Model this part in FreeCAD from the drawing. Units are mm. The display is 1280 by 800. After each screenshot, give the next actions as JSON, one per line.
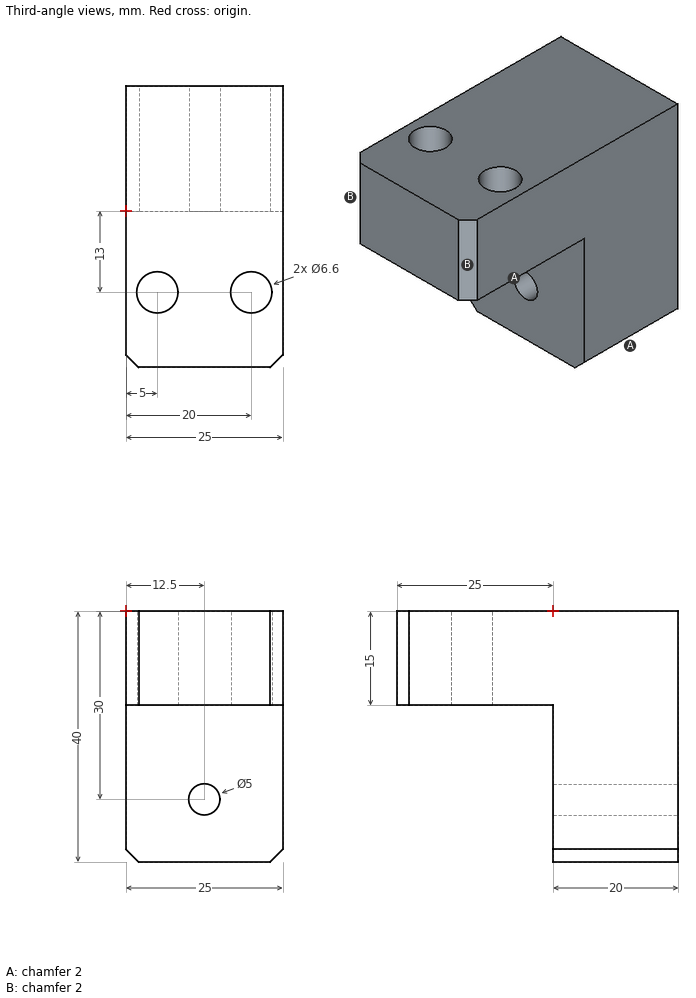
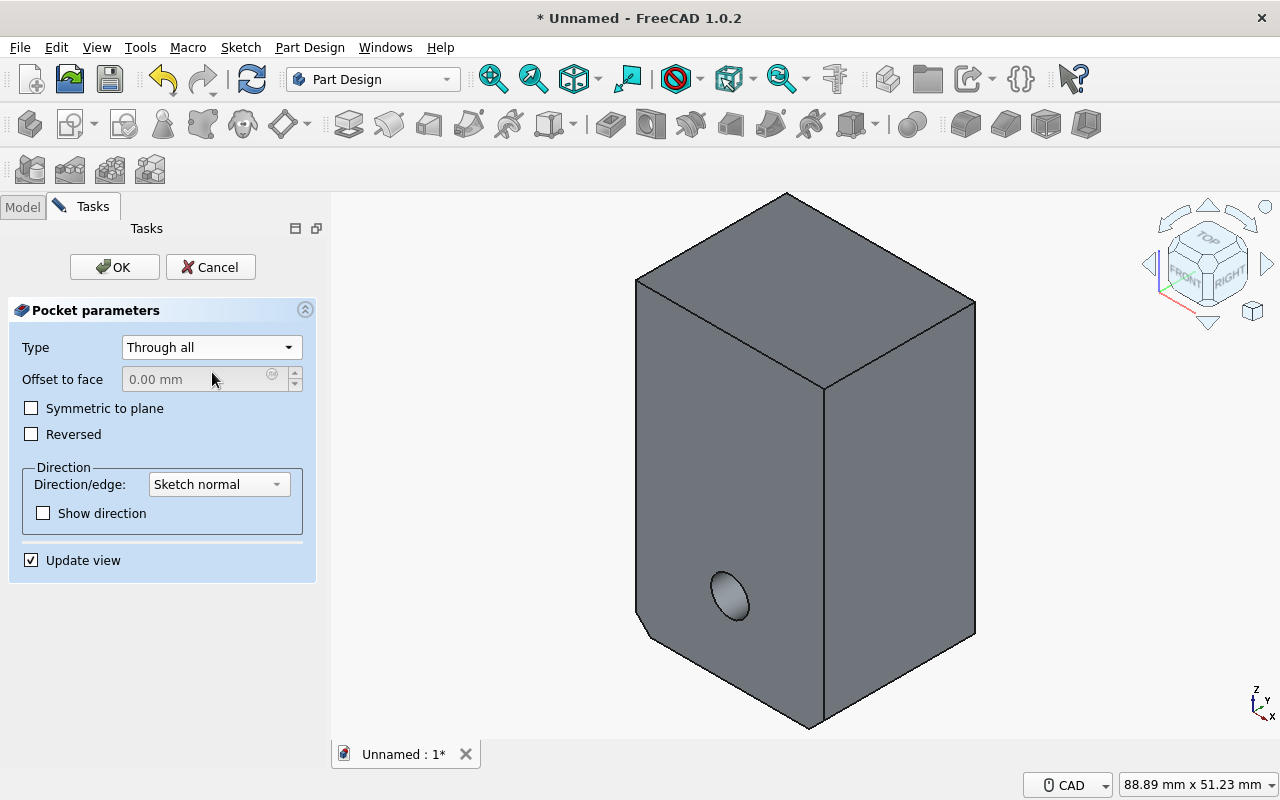
{"action": "left_click", "coordinate": [115, 267]}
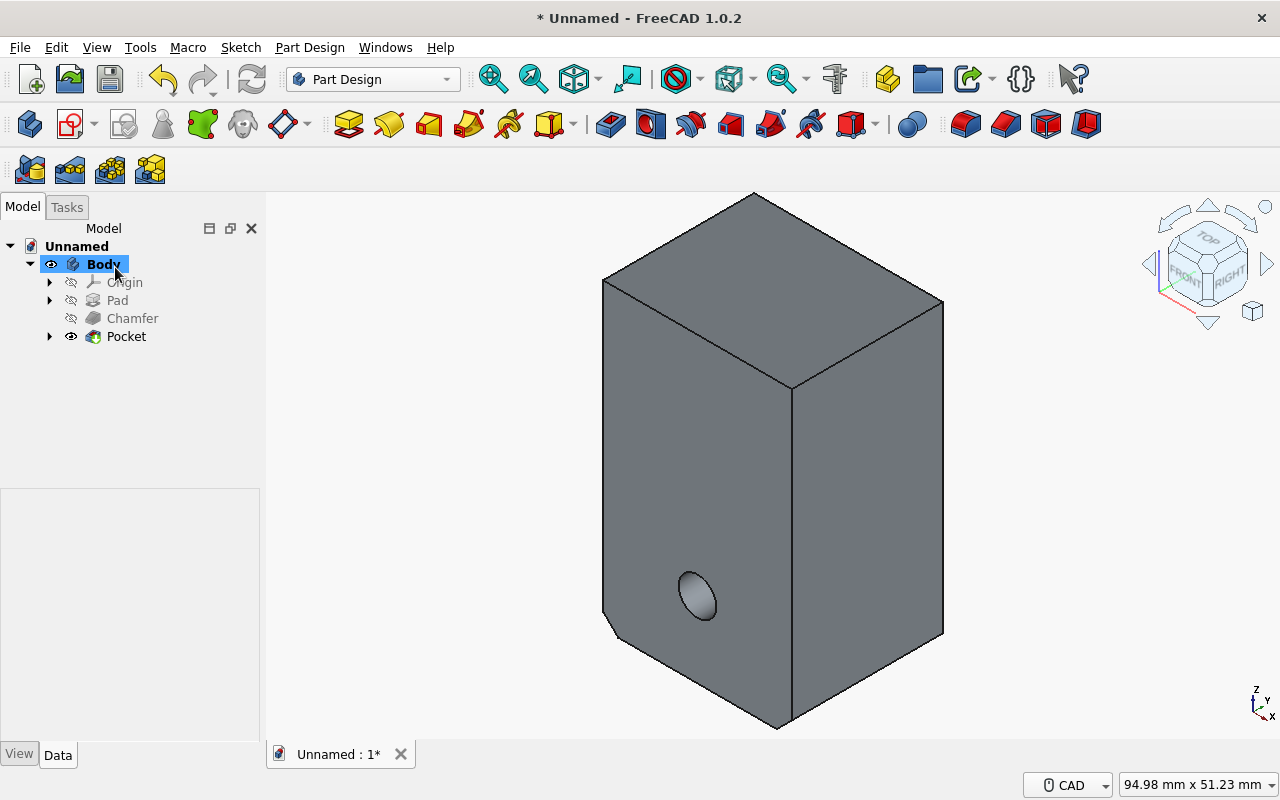
{"action": "left_click", "coordinate": [867, 463]}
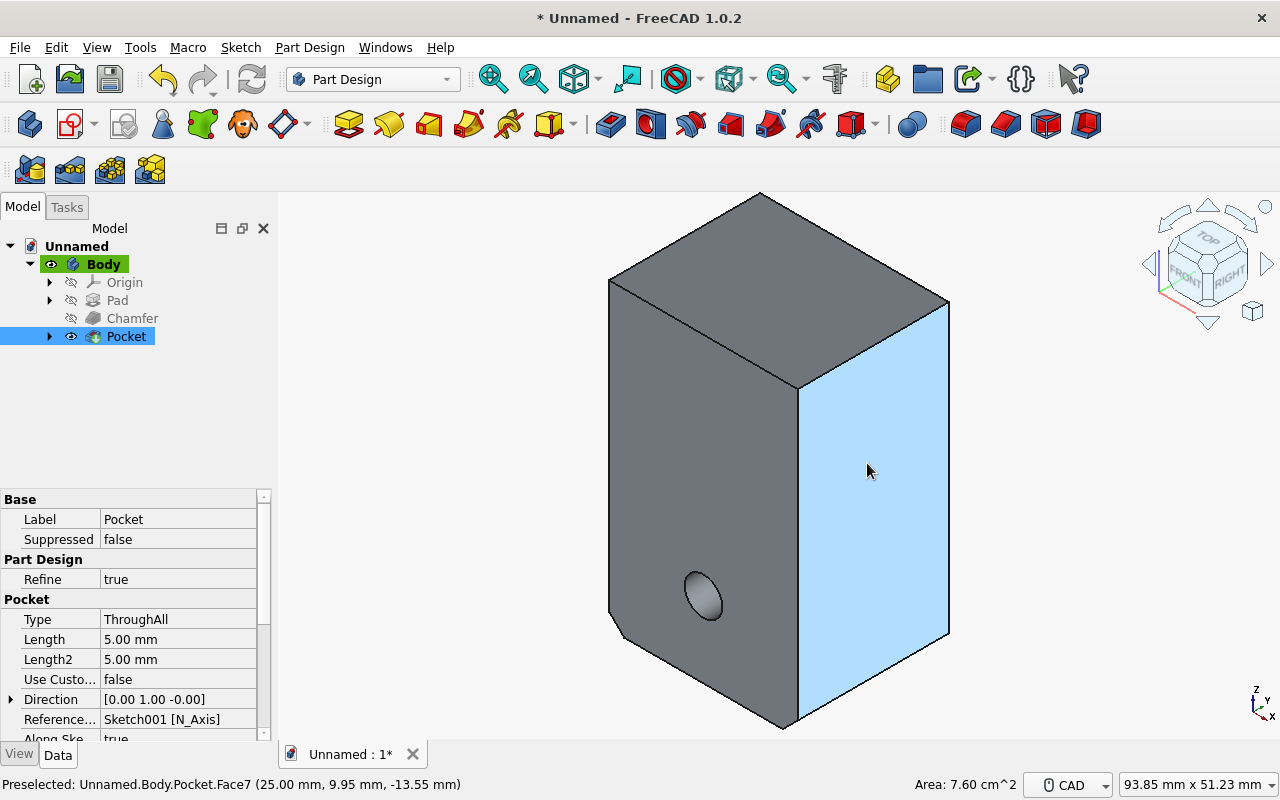
{"action": "left_click", "coordinate": [70, 124]}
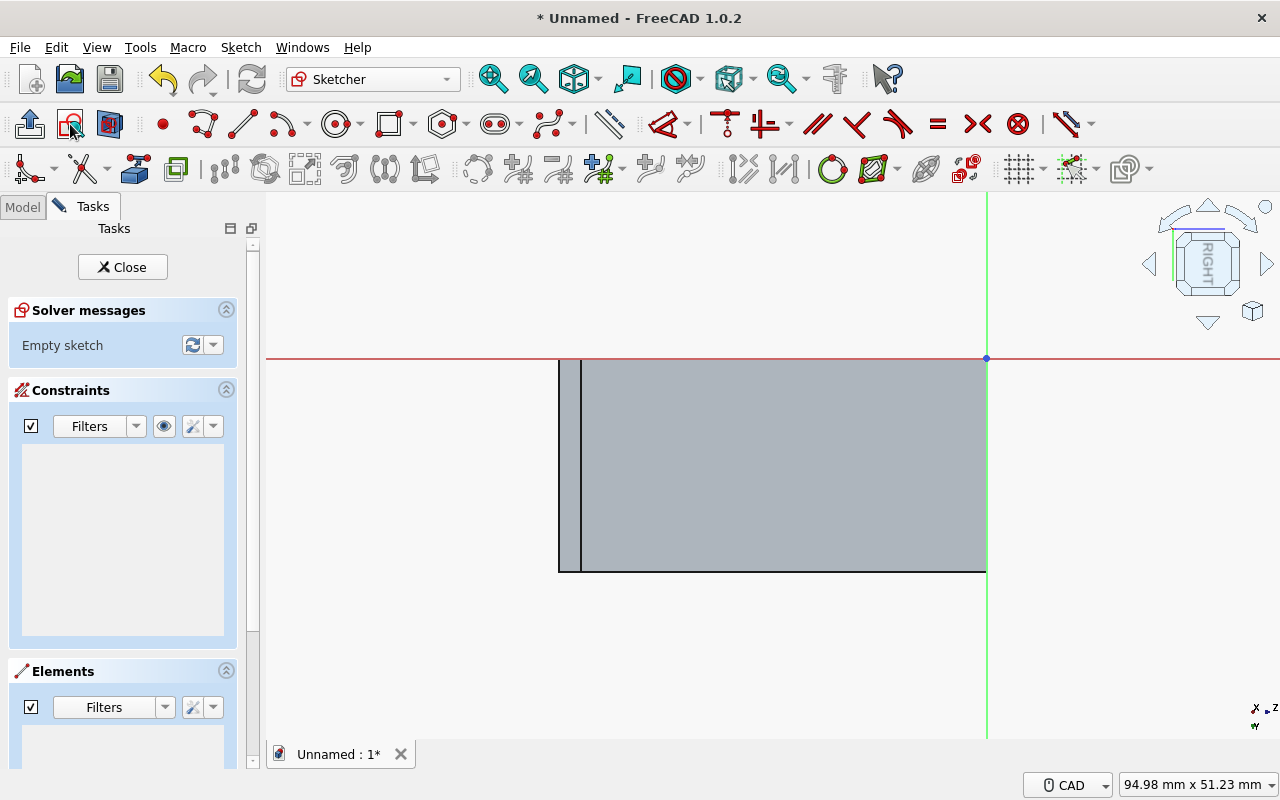
{"action": "scroll", "coordinate": [294, 711], "scroll_direction": "down", "scroll_amount": 2}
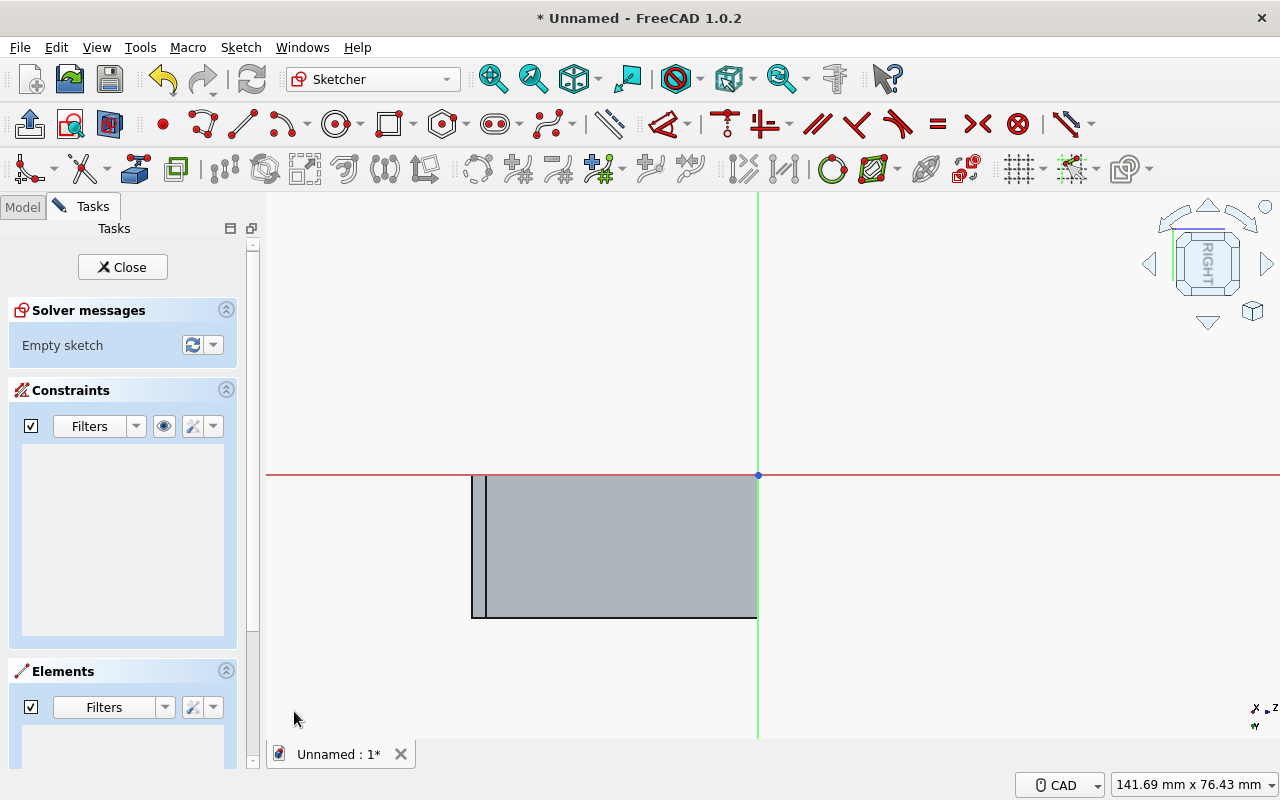
{"action": "scroll", "coordinate": [705, 289], "scroll_direction": "up", "scroll_amount": 3}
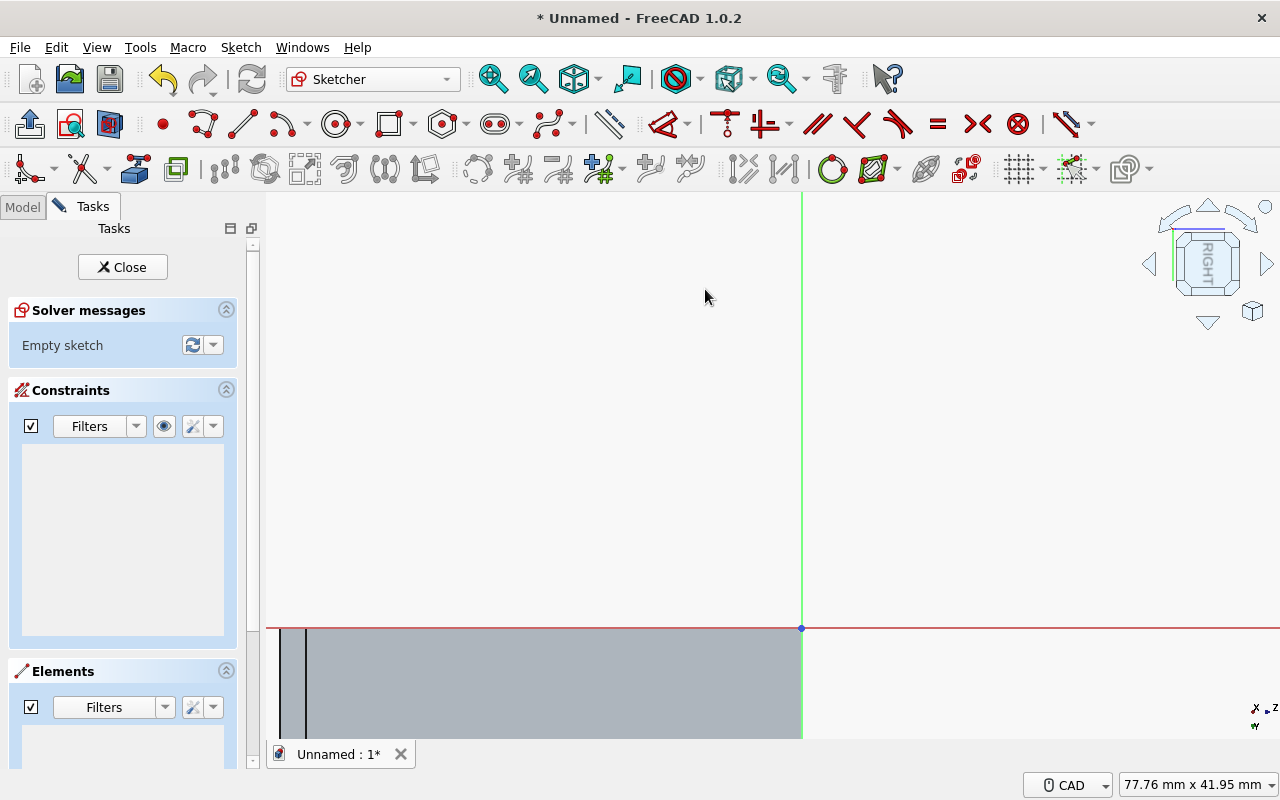
{"action": "key", "text": "g r"}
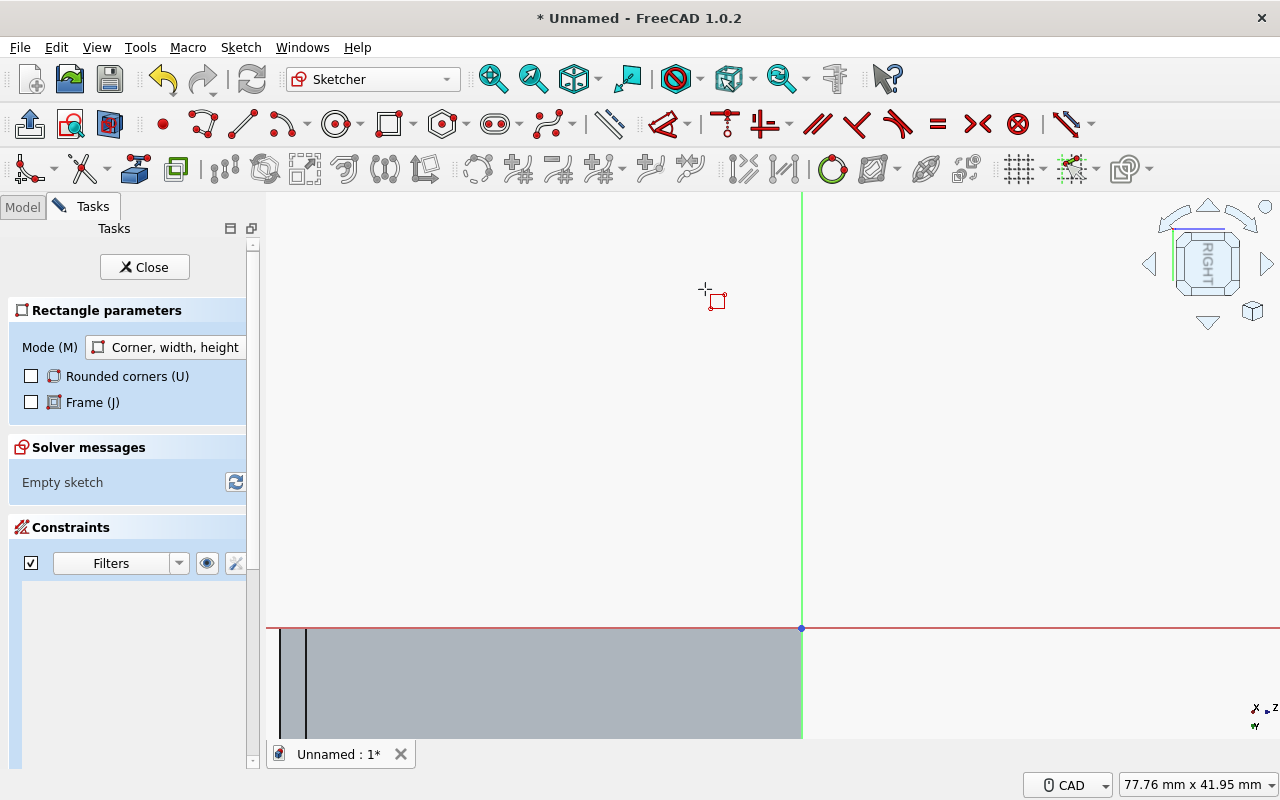
{"action": "left_click", "coordinate": [802, 628]}
{"action": "left_click", "coordinate": [606, 302]}
{"action": "key", "text": "Escape"}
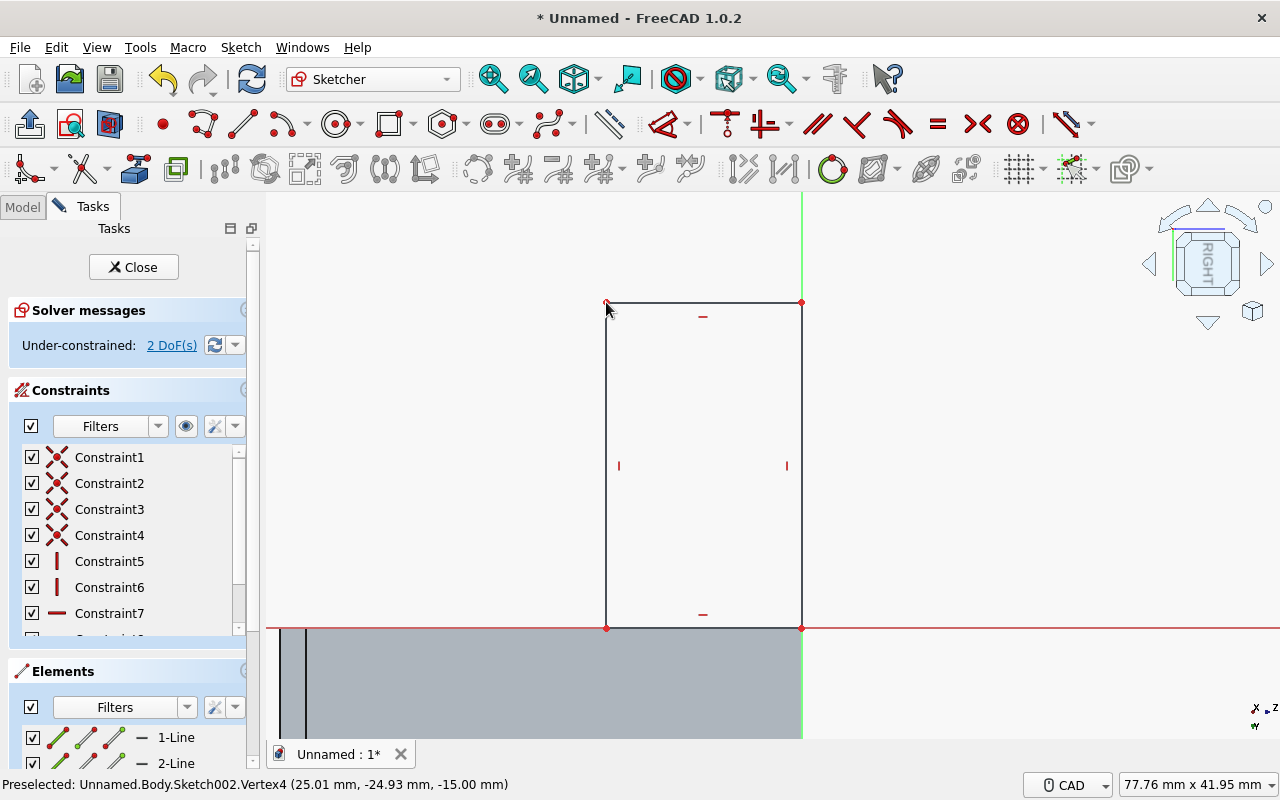
{"action": "left_click", "coordinate": [802, 531]}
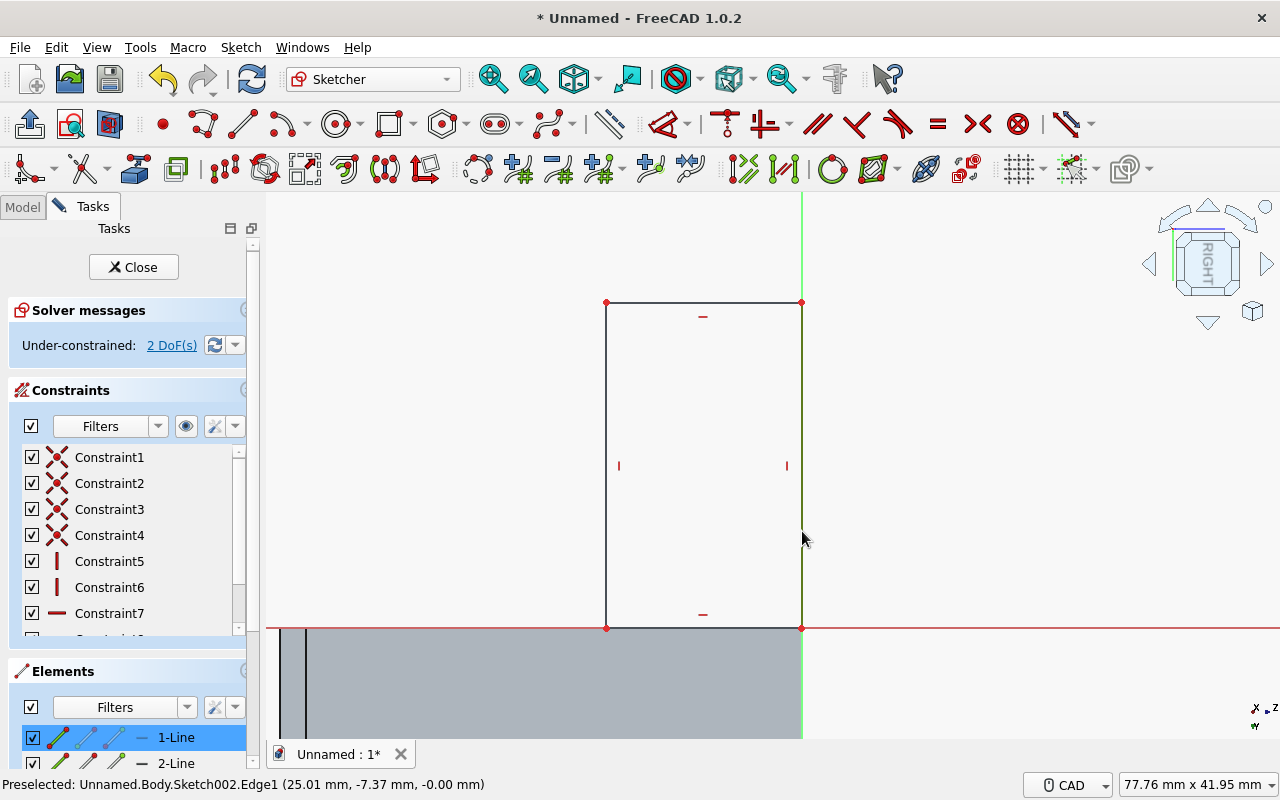
{"action": "key", "text": "i"}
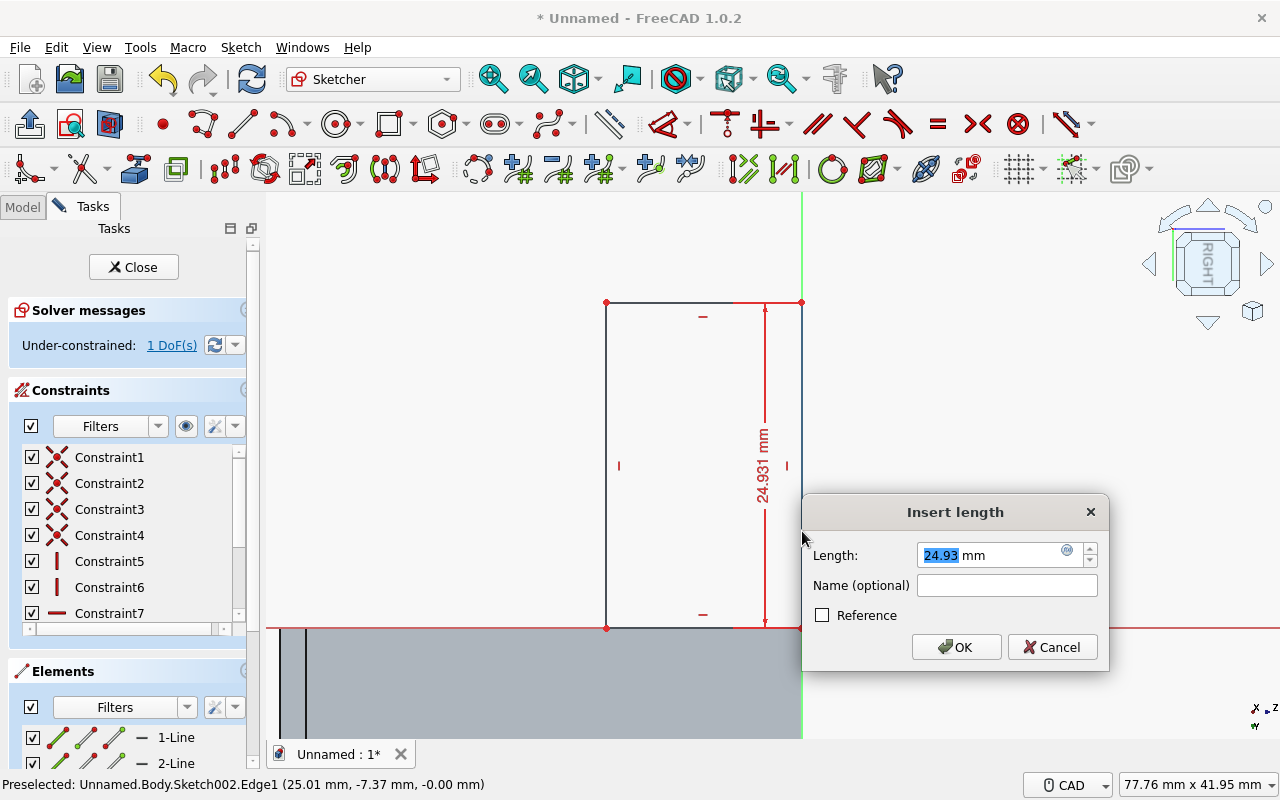
{"action": "type", "text": "25"}
{"action": "key", "text": "Return"}